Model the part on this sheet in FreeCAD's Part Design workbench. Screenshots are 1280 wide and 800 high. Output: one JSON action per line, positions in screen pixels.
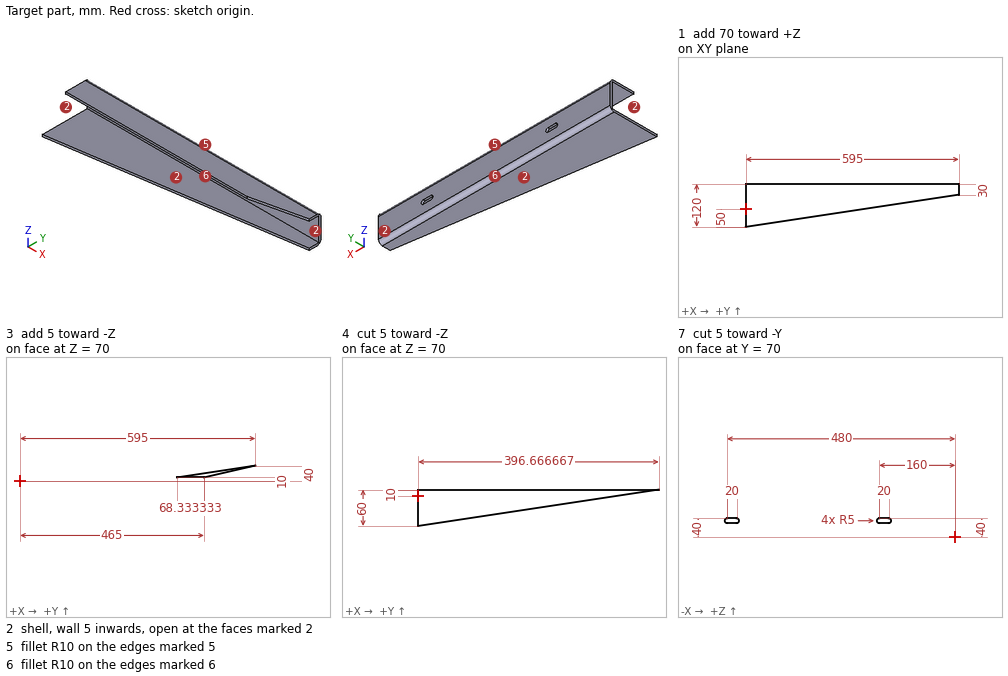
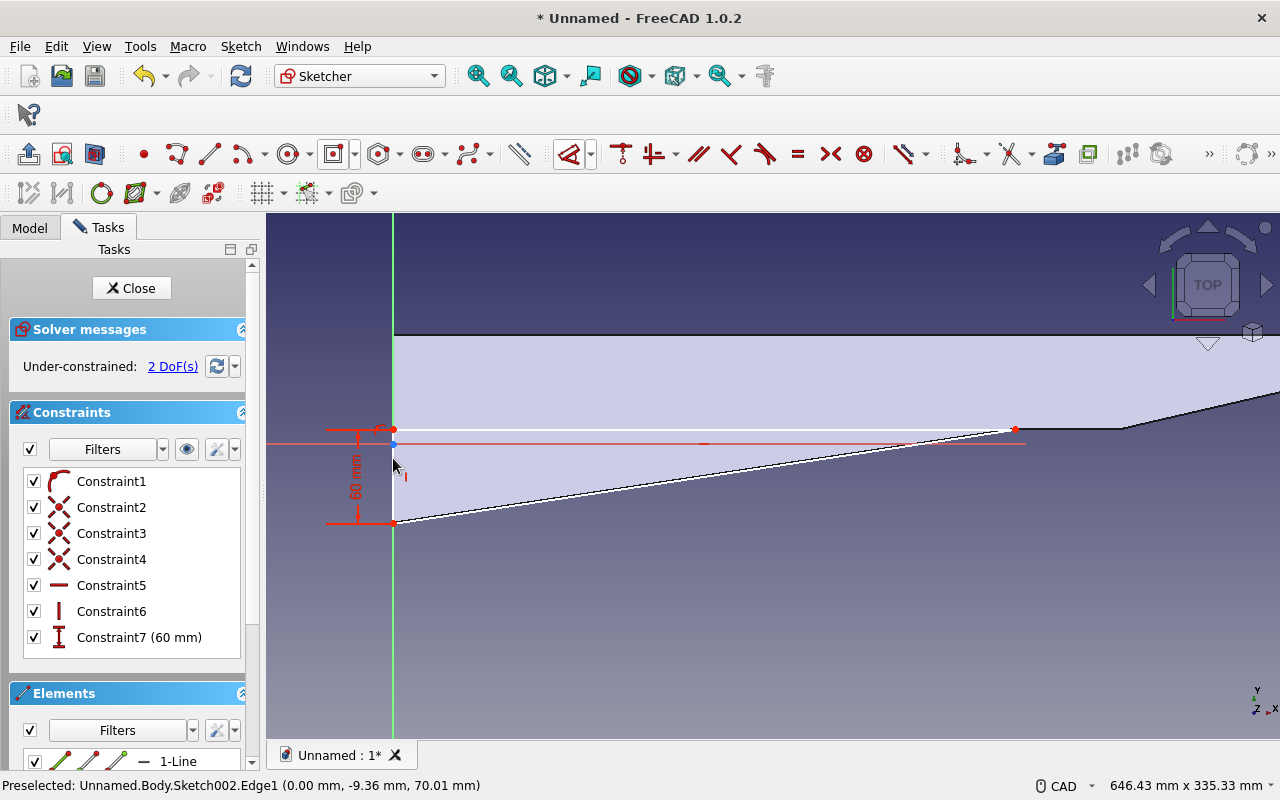
{"action": "scroll", "coordinate": [393, 430], "scroll_direction": "up", "scroll_amount": 5}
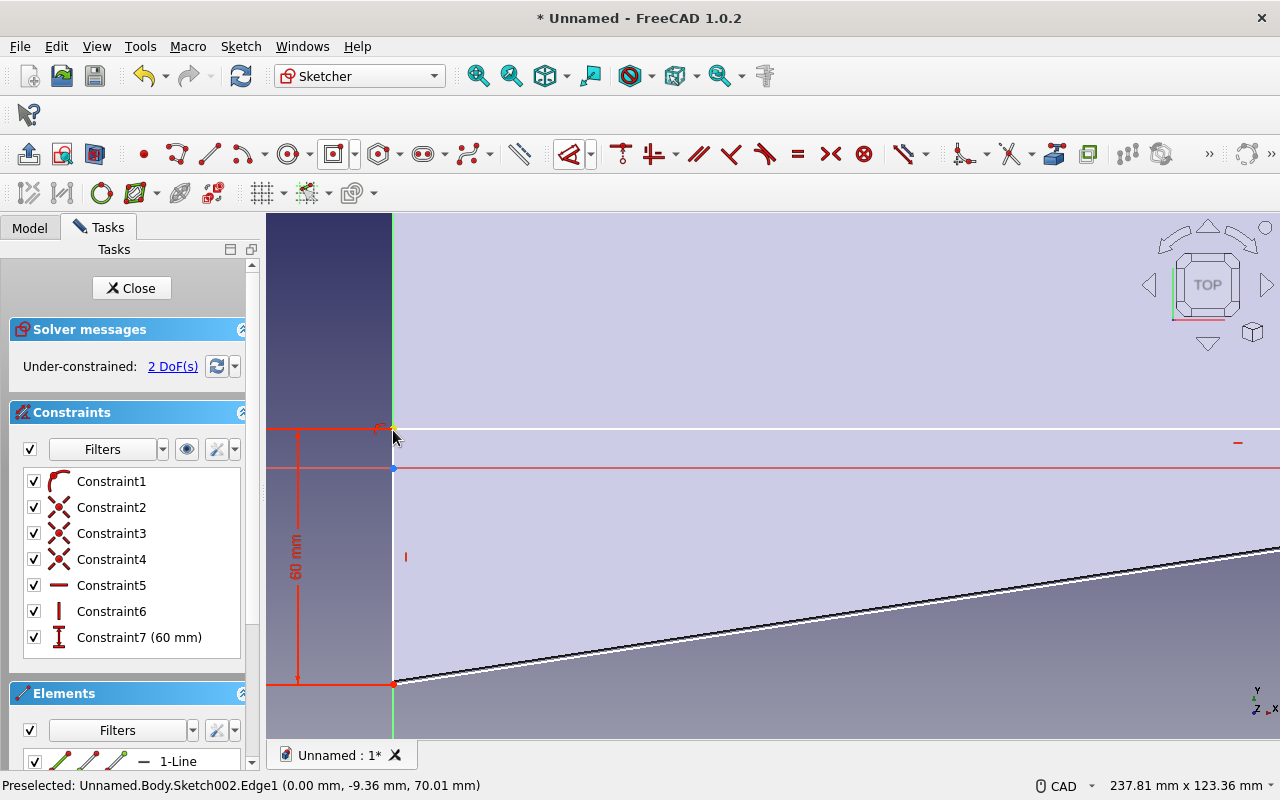
{"action": "left_click", "coordinate": [393, 429]}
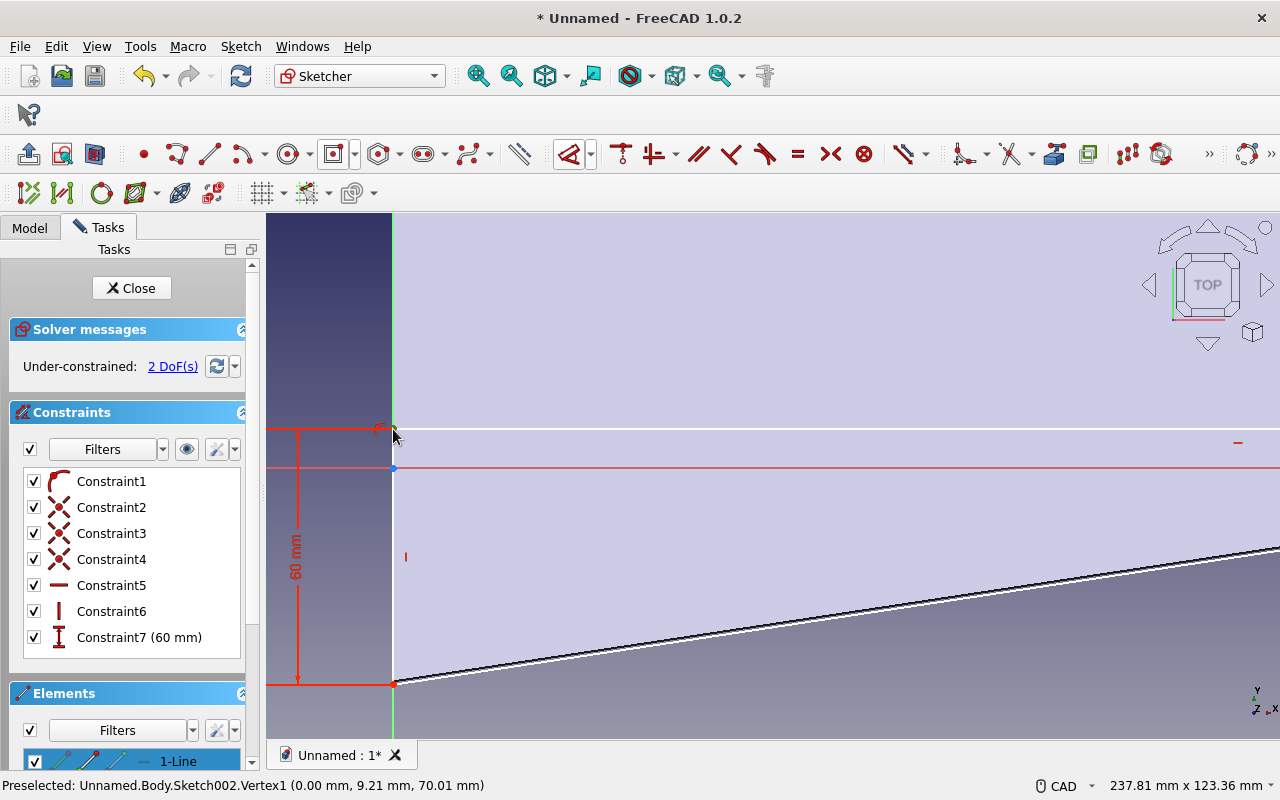
{"action": "left_click", "coordinate": [590, 154]}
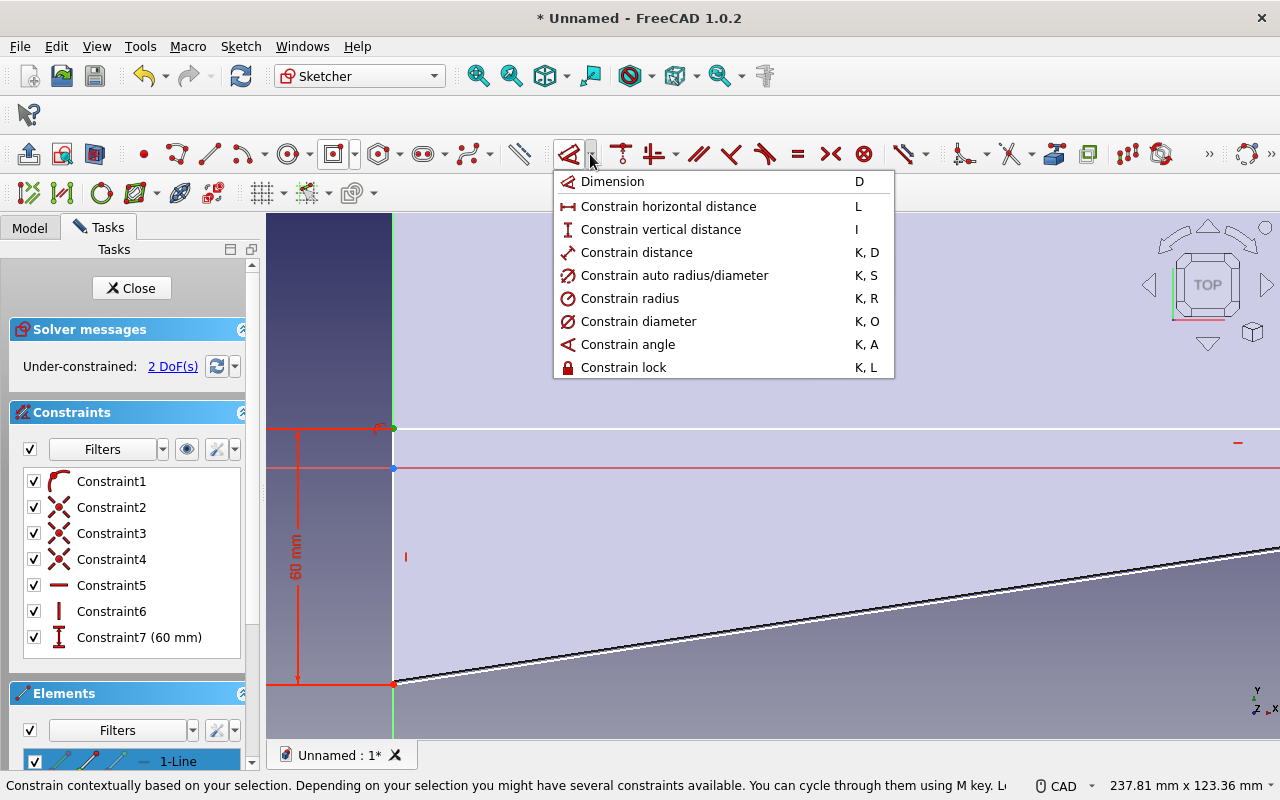
{"action": "left_click", "coordinate": [724, 230]}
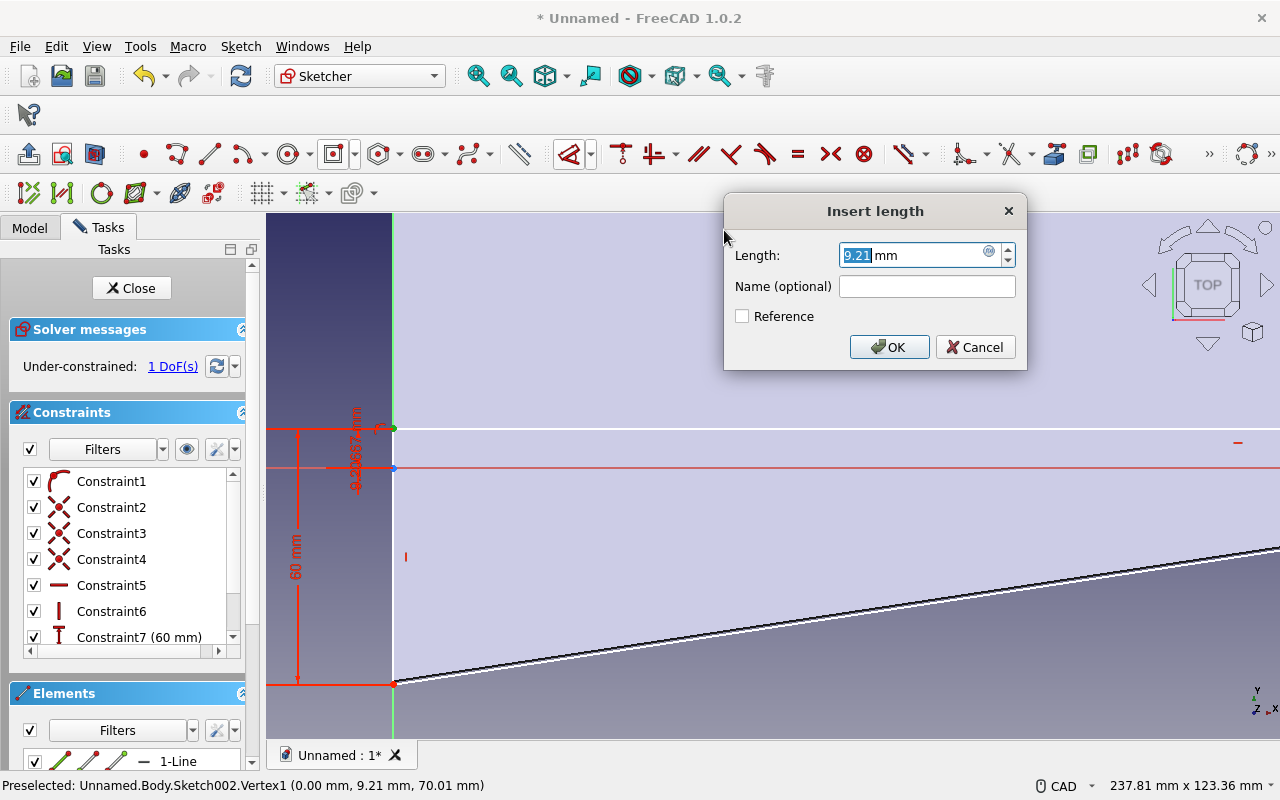
{"action": "type", "text": "10"}
{"action": "key", "text": "Return"}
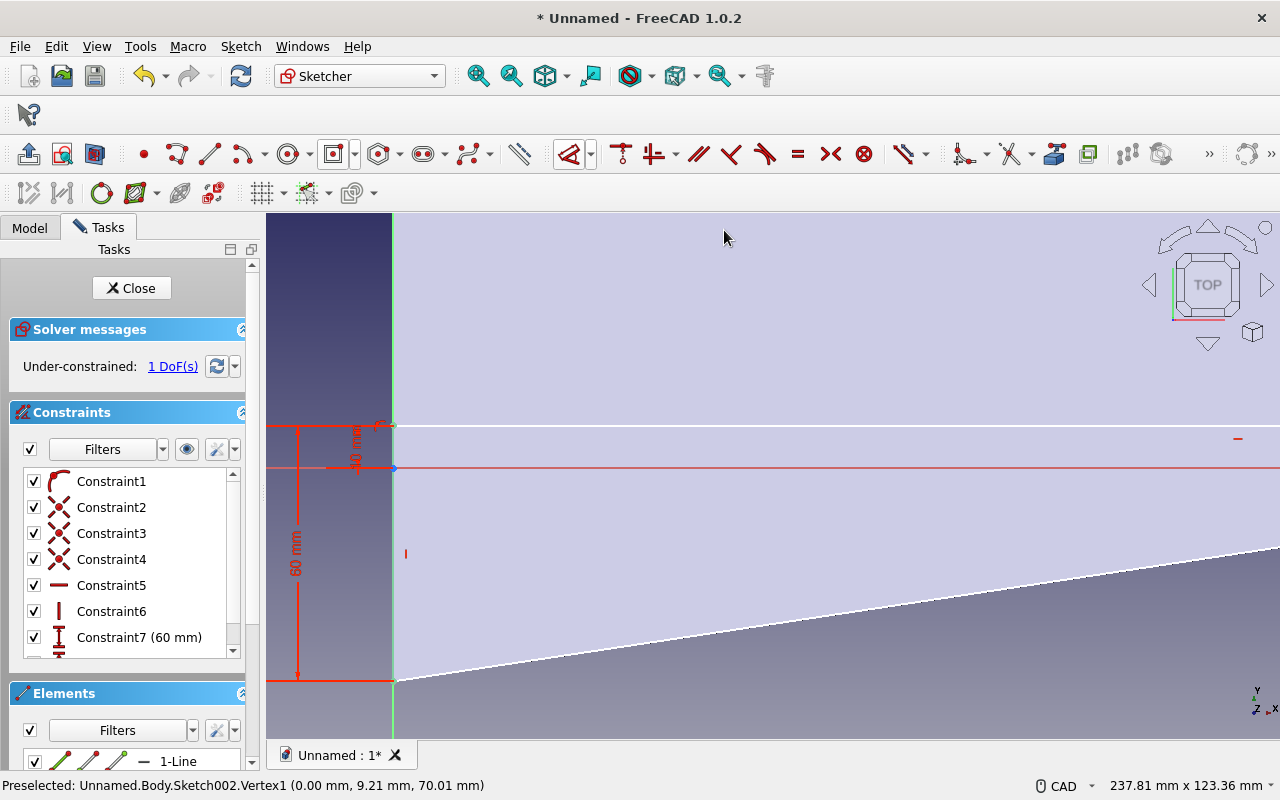
{"action": "left_click", "coordinate": [900, 426]}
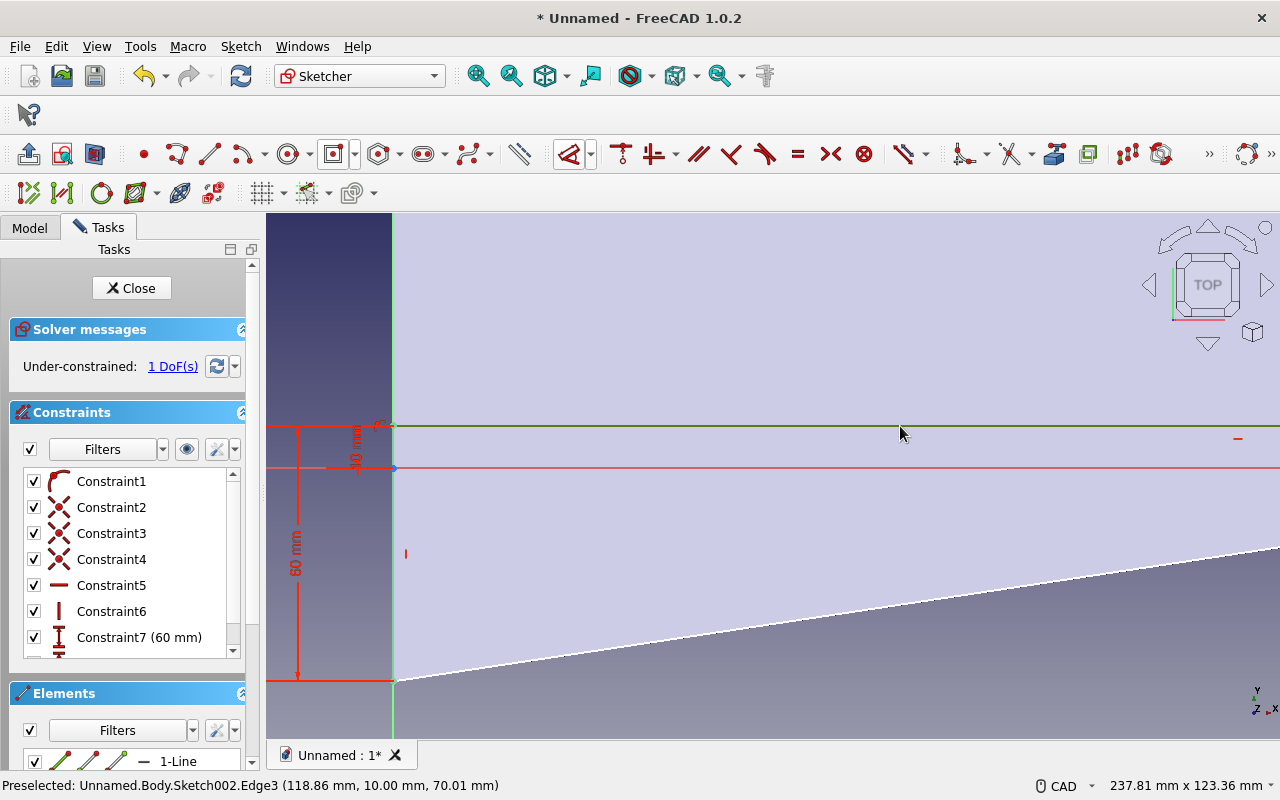
{"action": "key", "text": "l"}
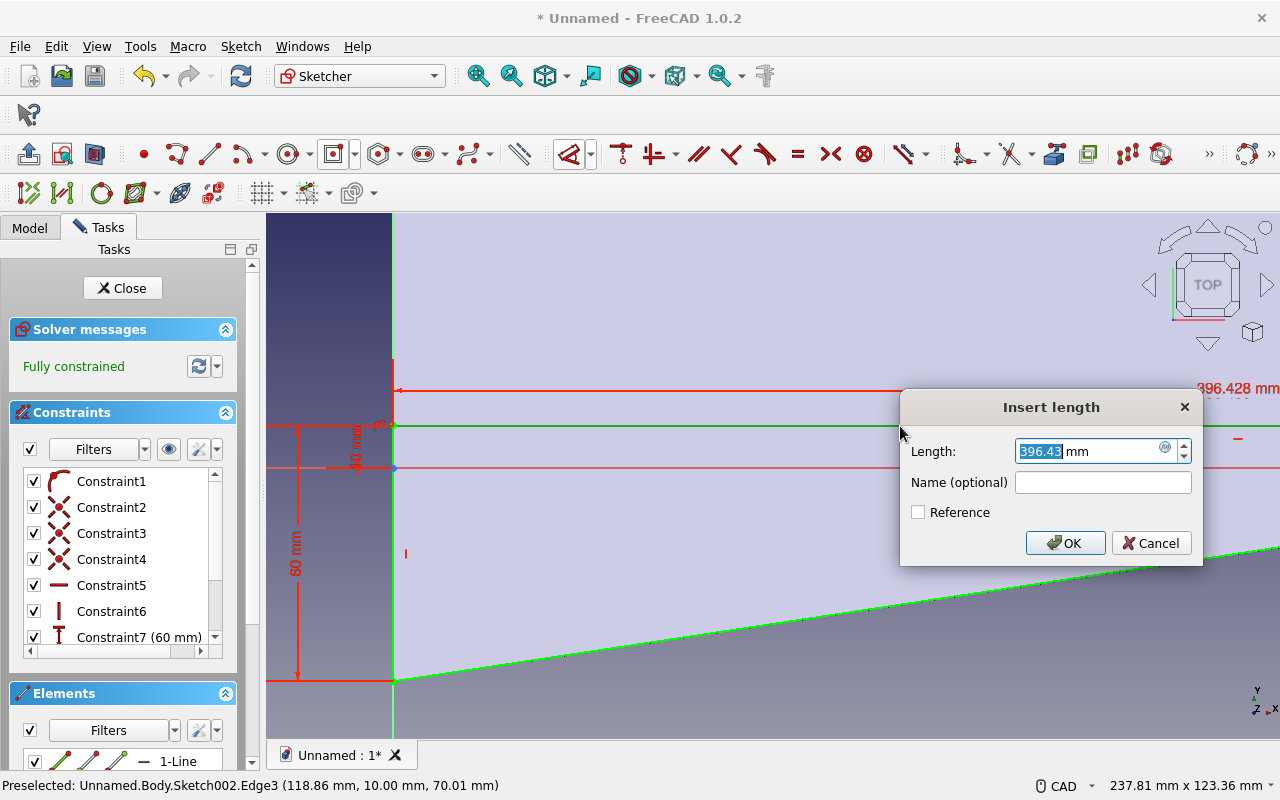
{"action": "type", "text": "396.666667"}
{"action": "key", "text": "Return"}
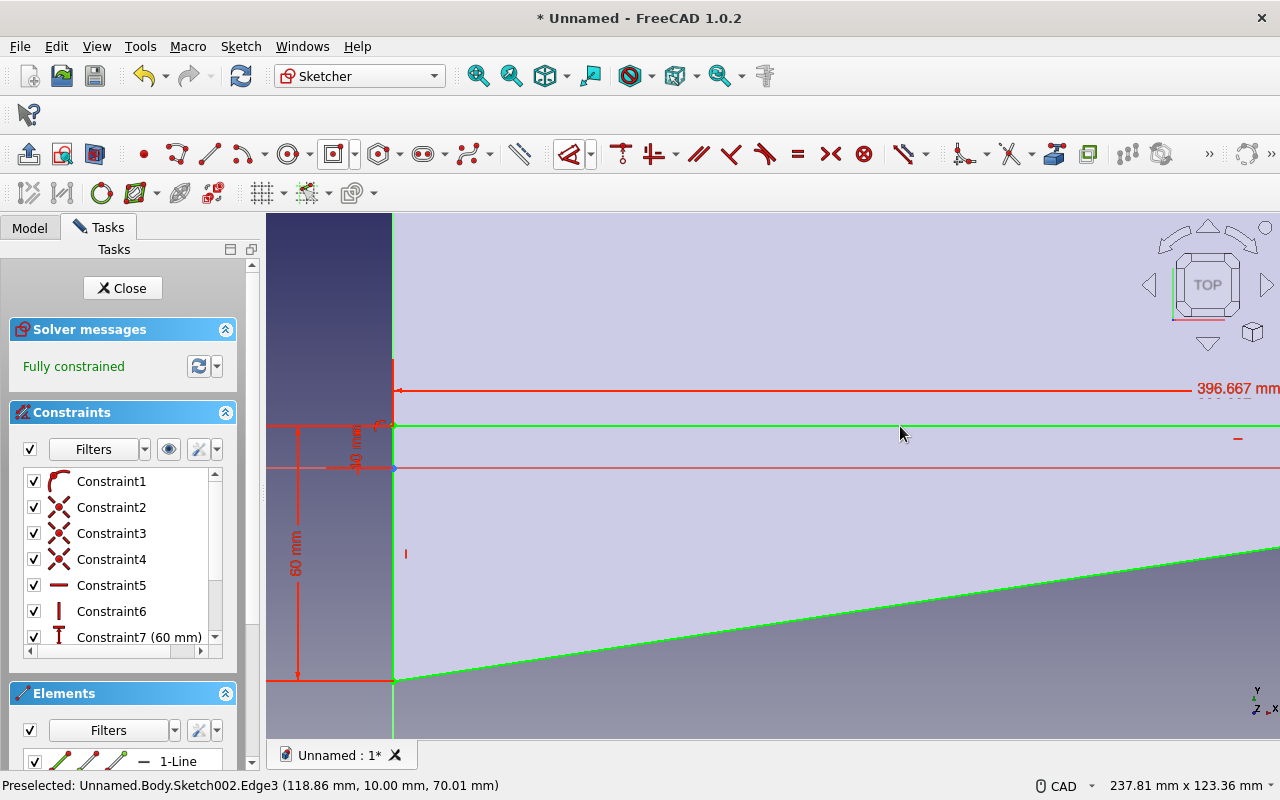
{"action": "left_click", "coordinate": [123, 288]}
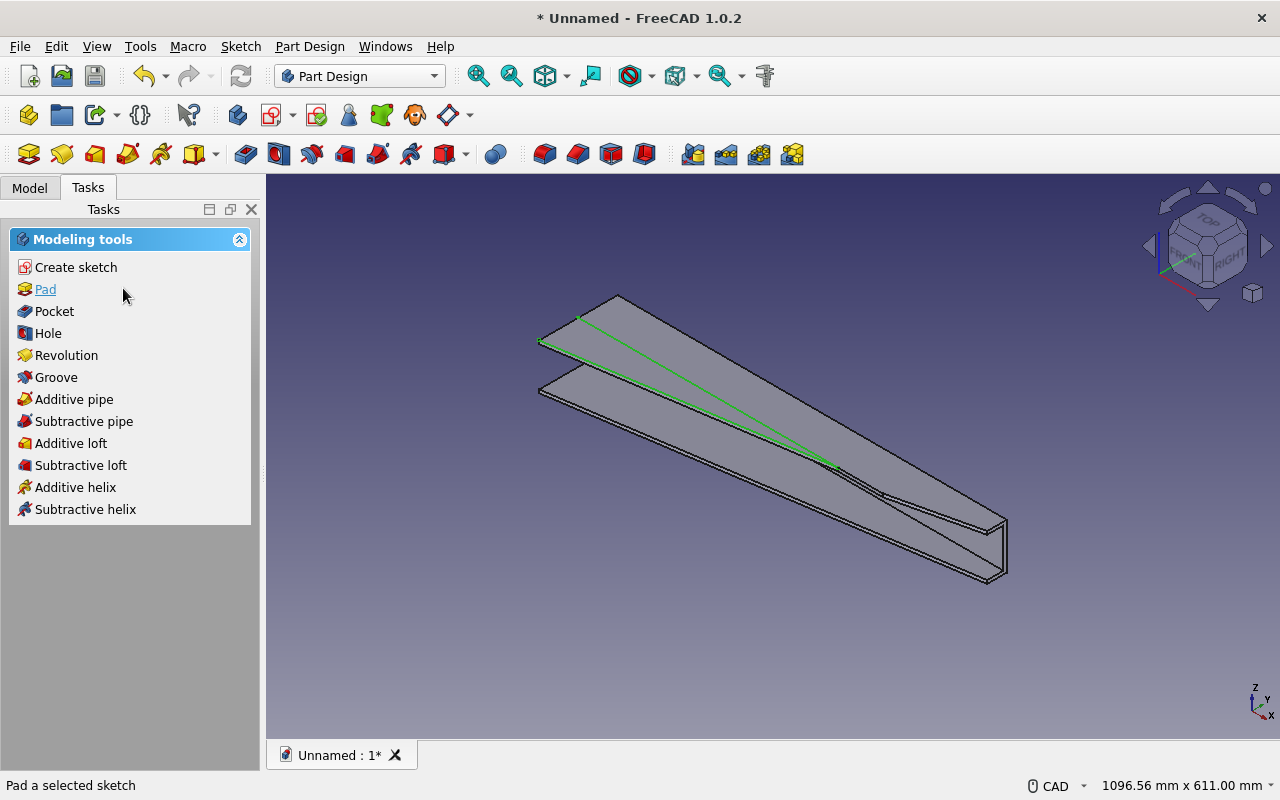
{"action": "left_click", "coordinate": [246, 154]}